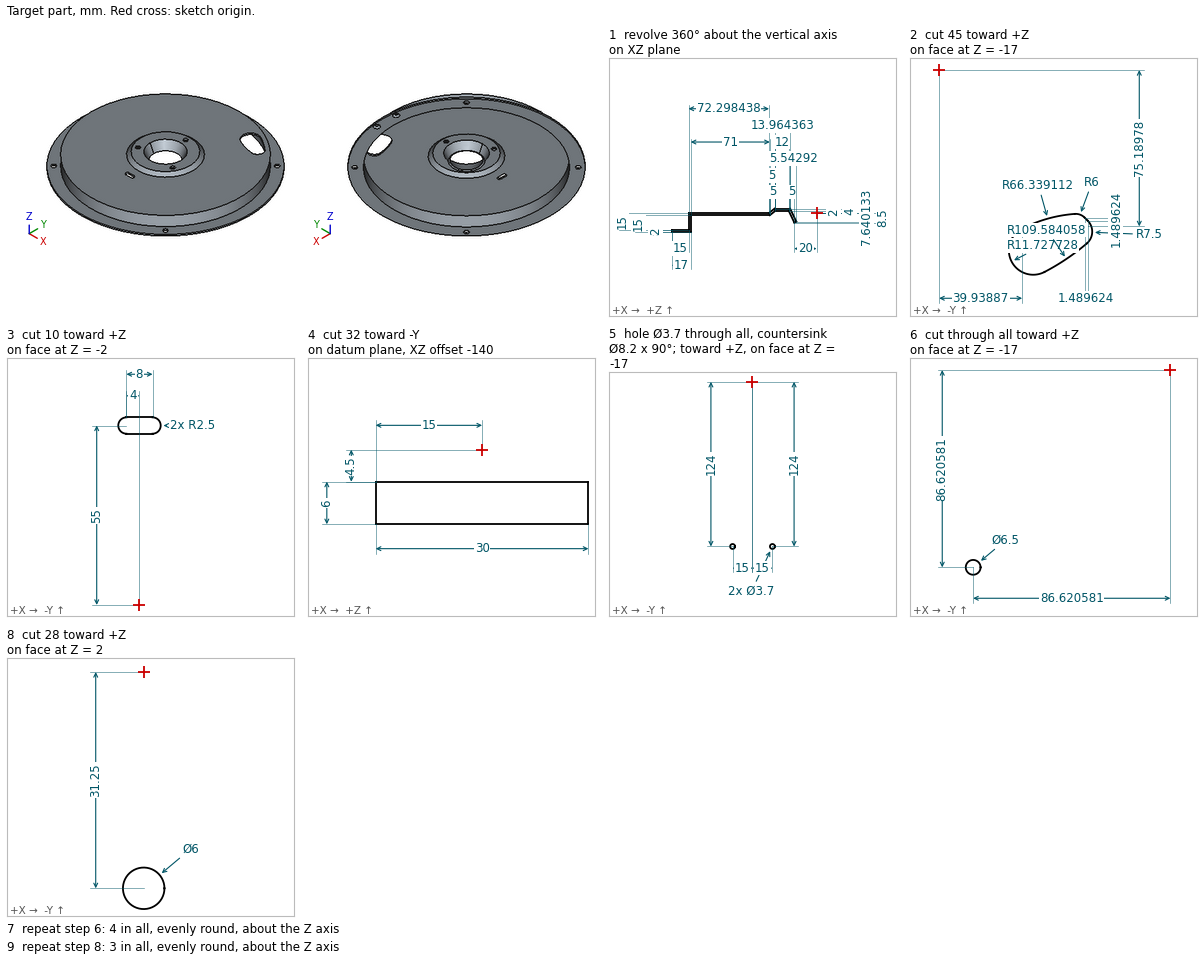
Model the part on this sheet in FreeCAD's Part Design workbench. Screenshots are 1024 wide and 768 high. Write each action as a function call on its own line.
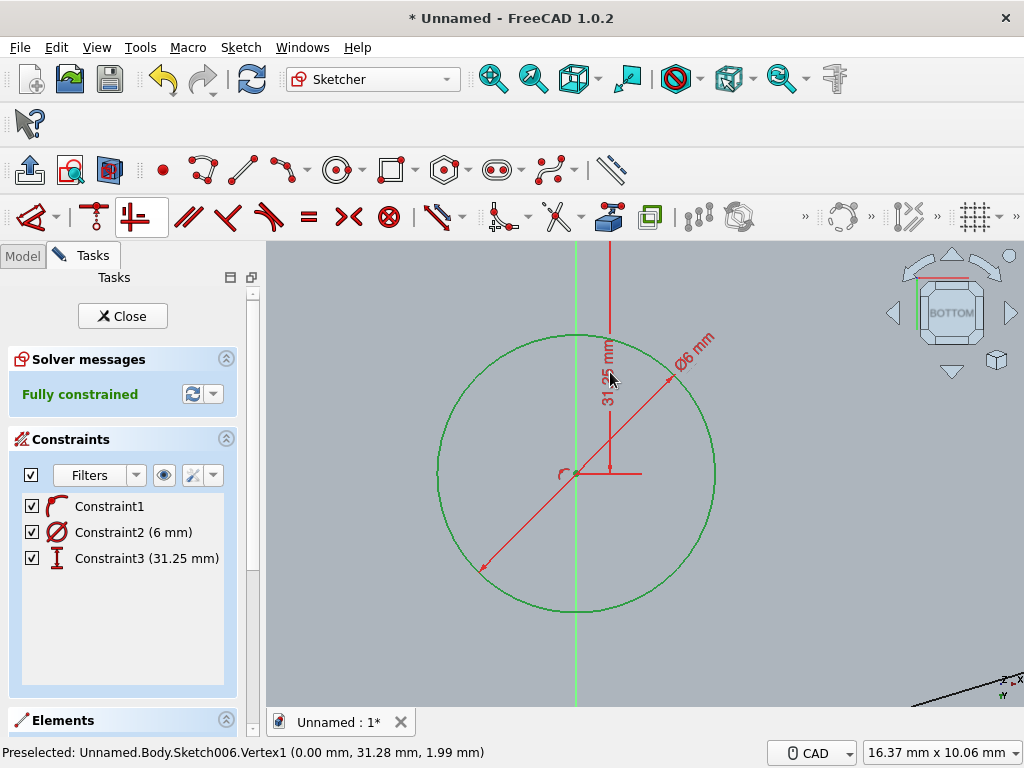
click(123, 316)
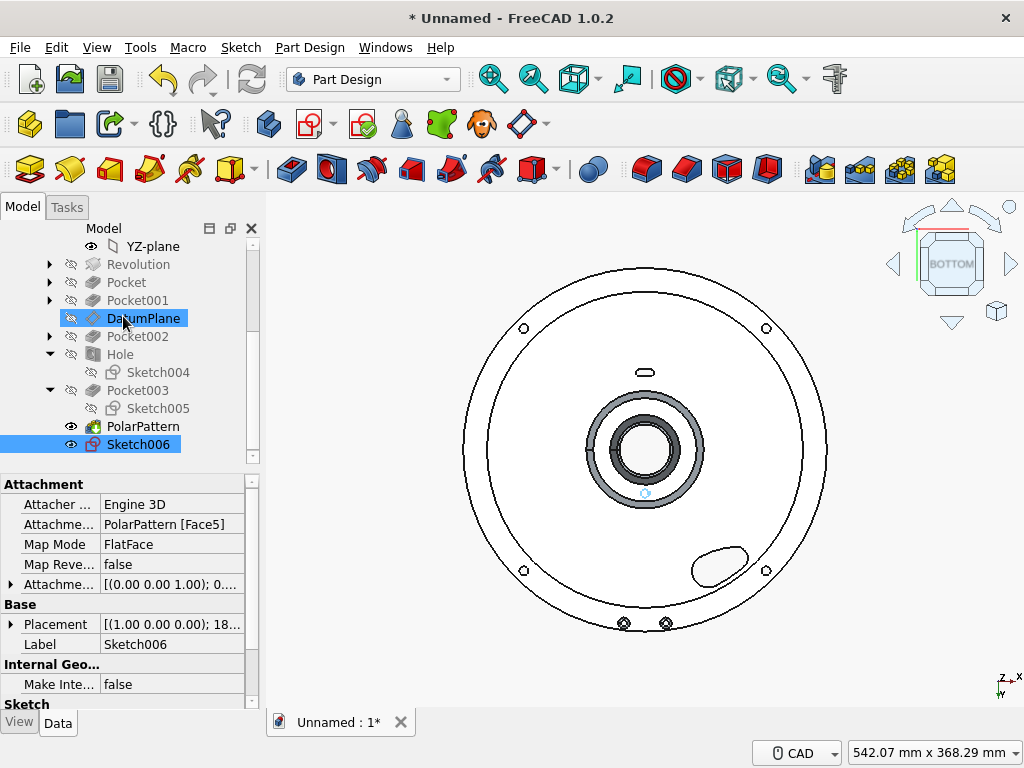
click(292, 170)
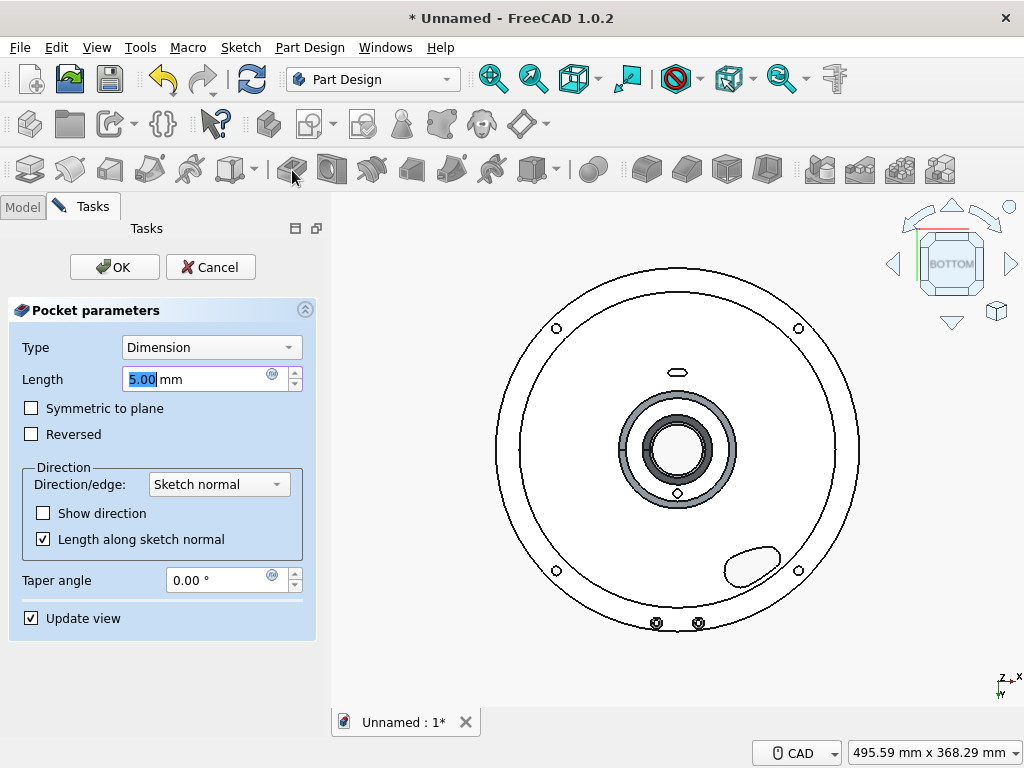
text(28)
key(Tab)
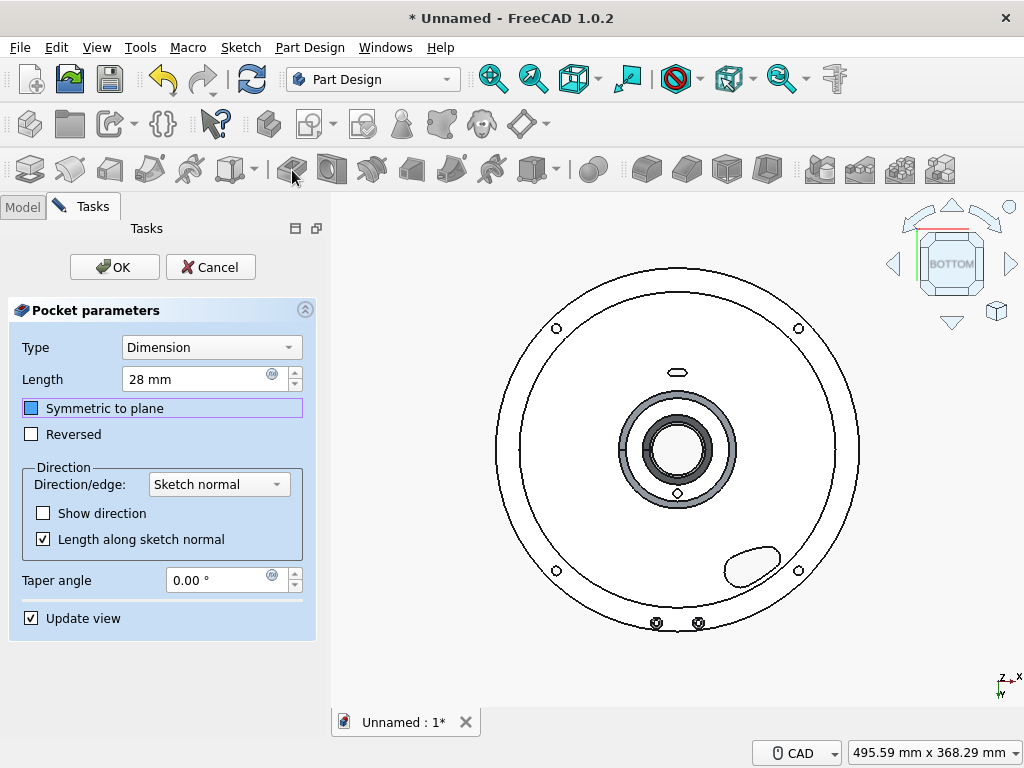
click(115, 267)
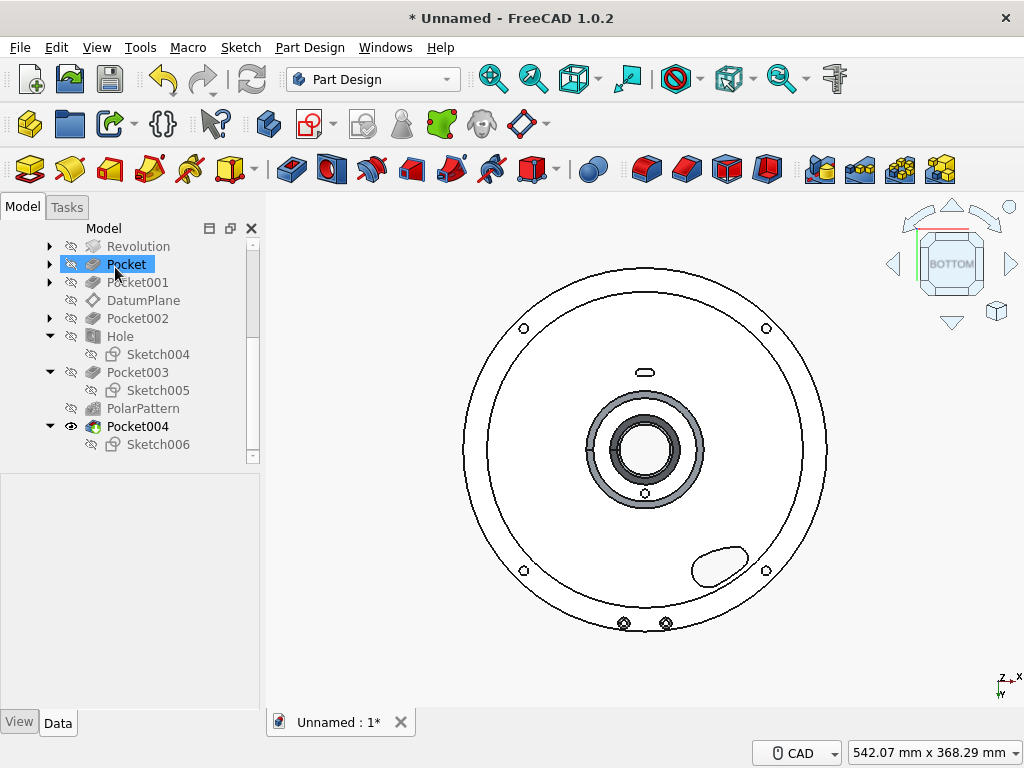
click(116, 426)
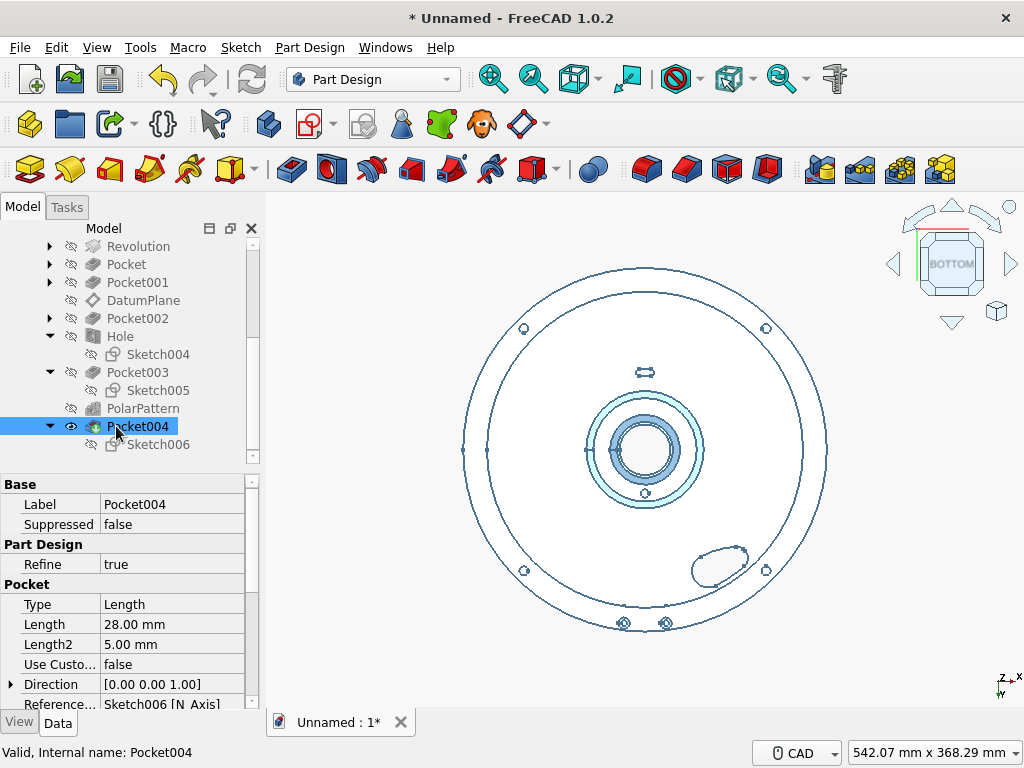
click(900, 170)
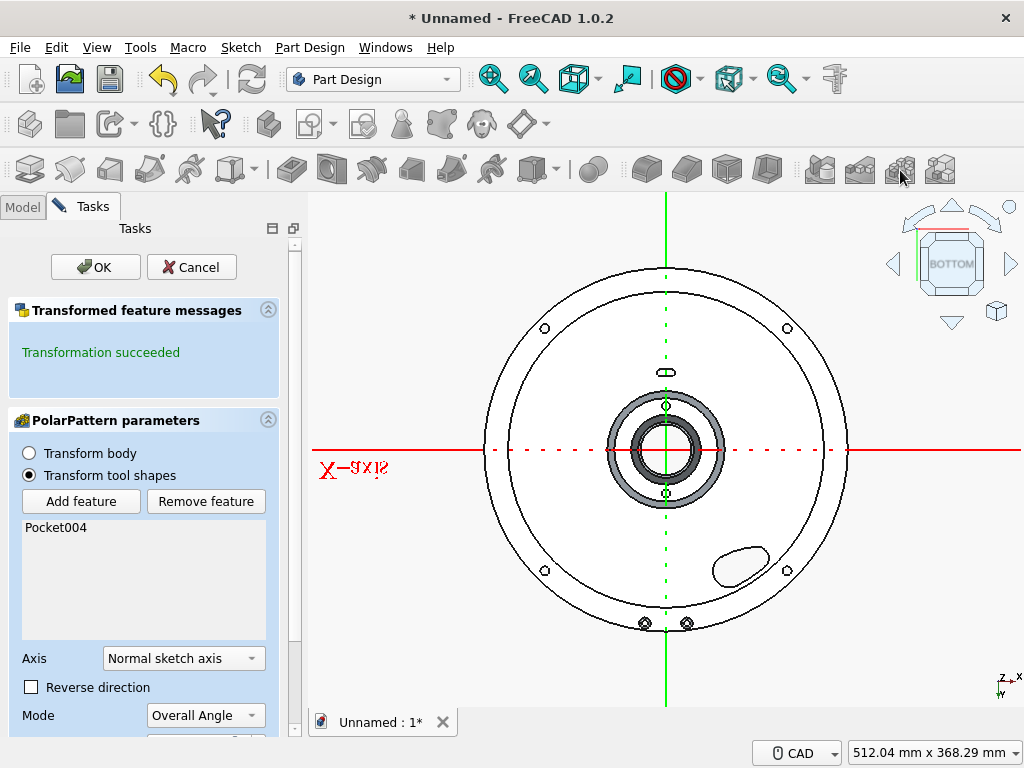
click(184, 658)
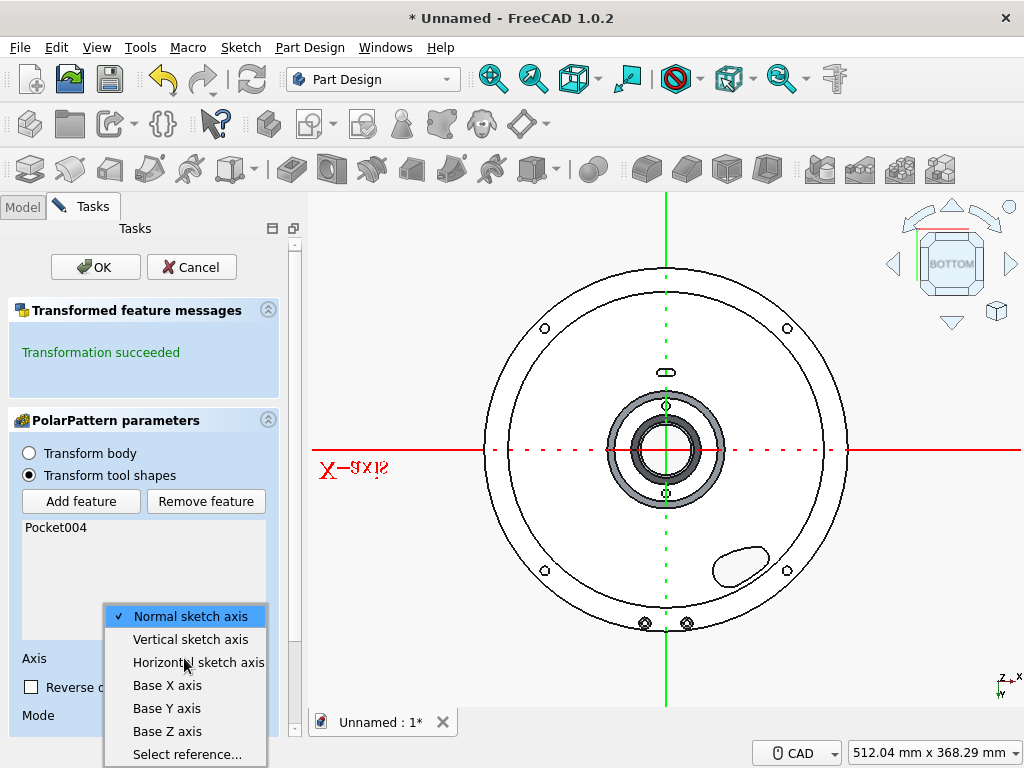
click(184, 732)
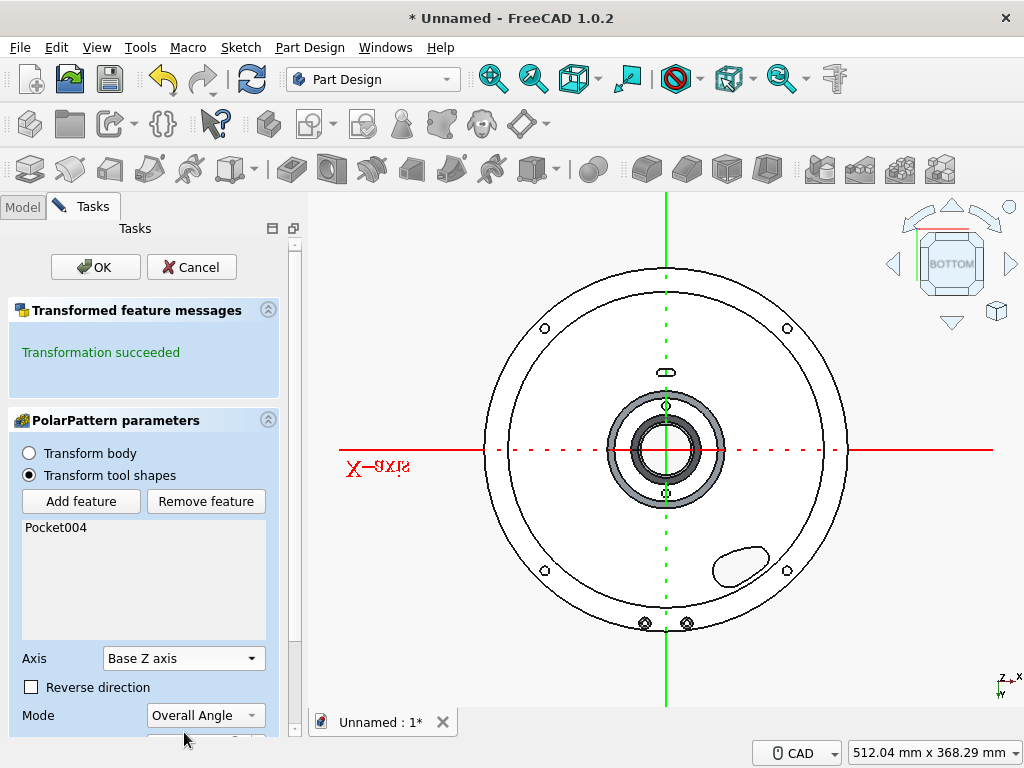
scroll(295, 487, down, 2)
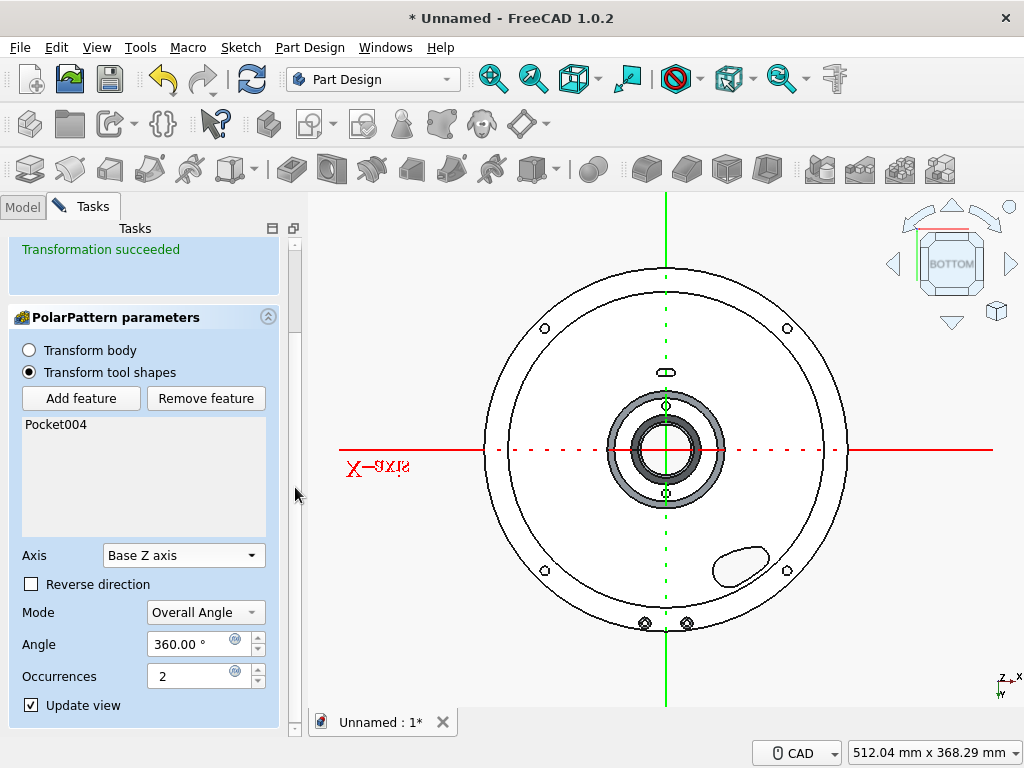
triple_click(198, 676)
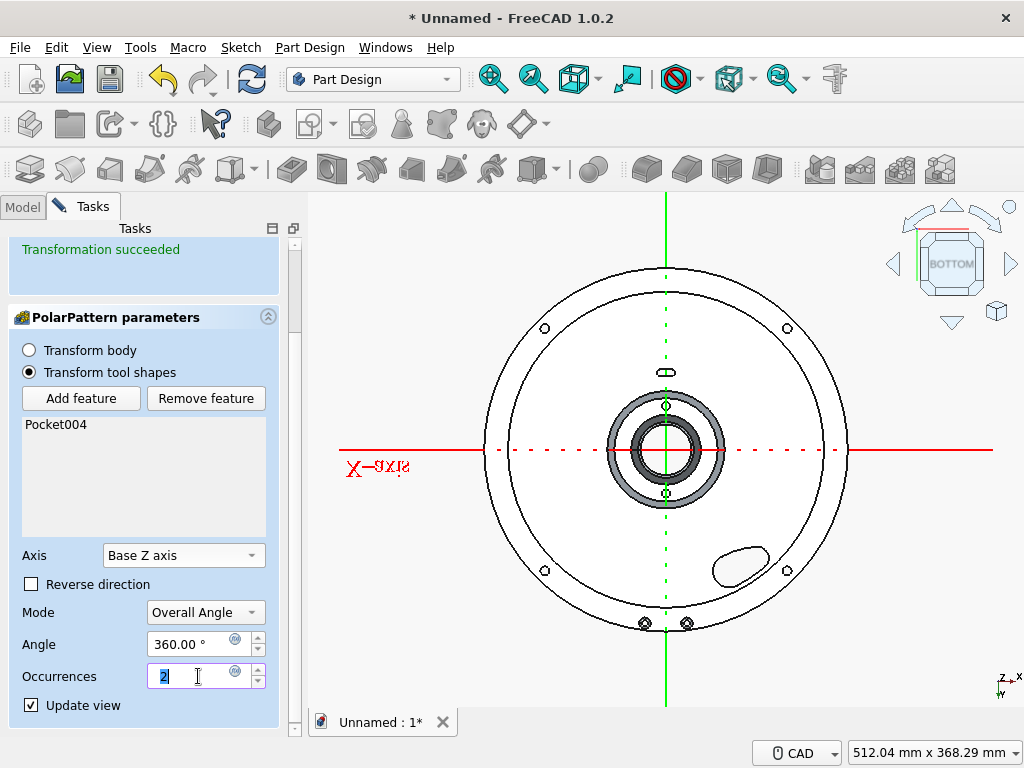
text(3)
key(Tab)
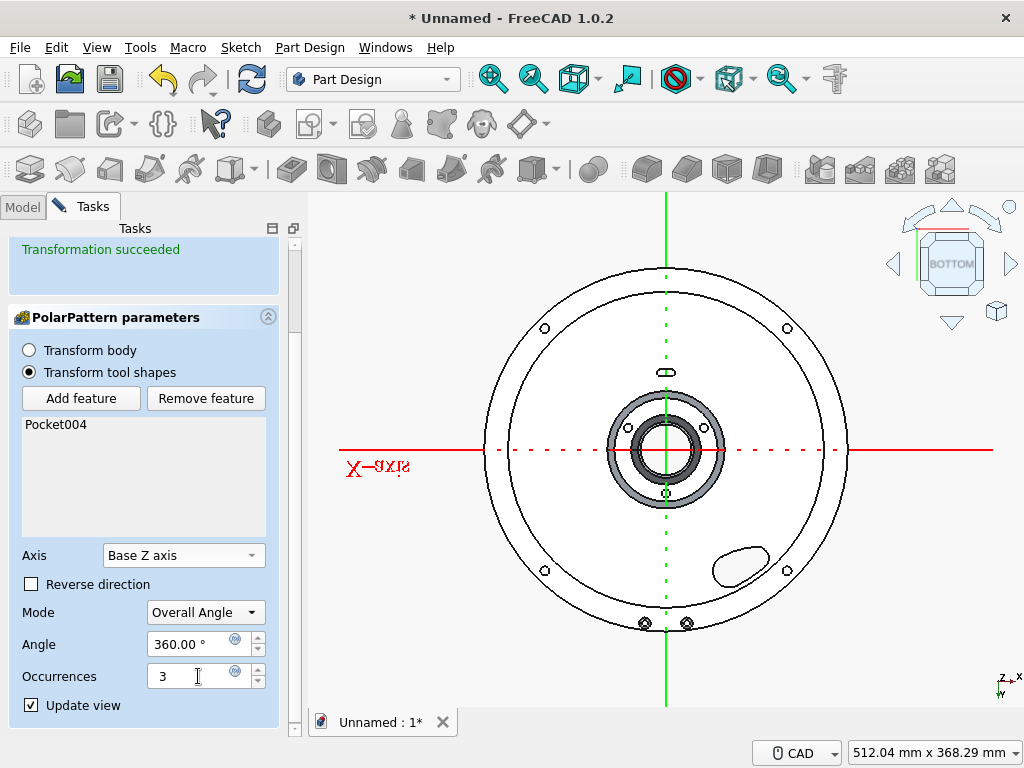
scroll(295, 487, up, 3)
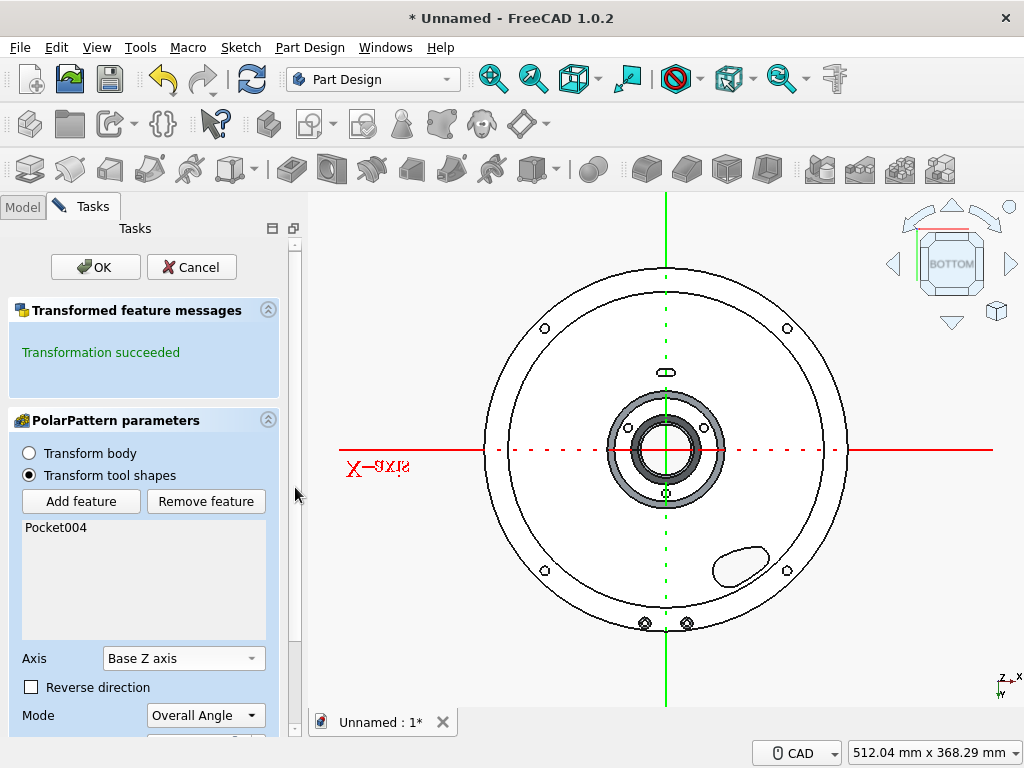
click(96, 267)